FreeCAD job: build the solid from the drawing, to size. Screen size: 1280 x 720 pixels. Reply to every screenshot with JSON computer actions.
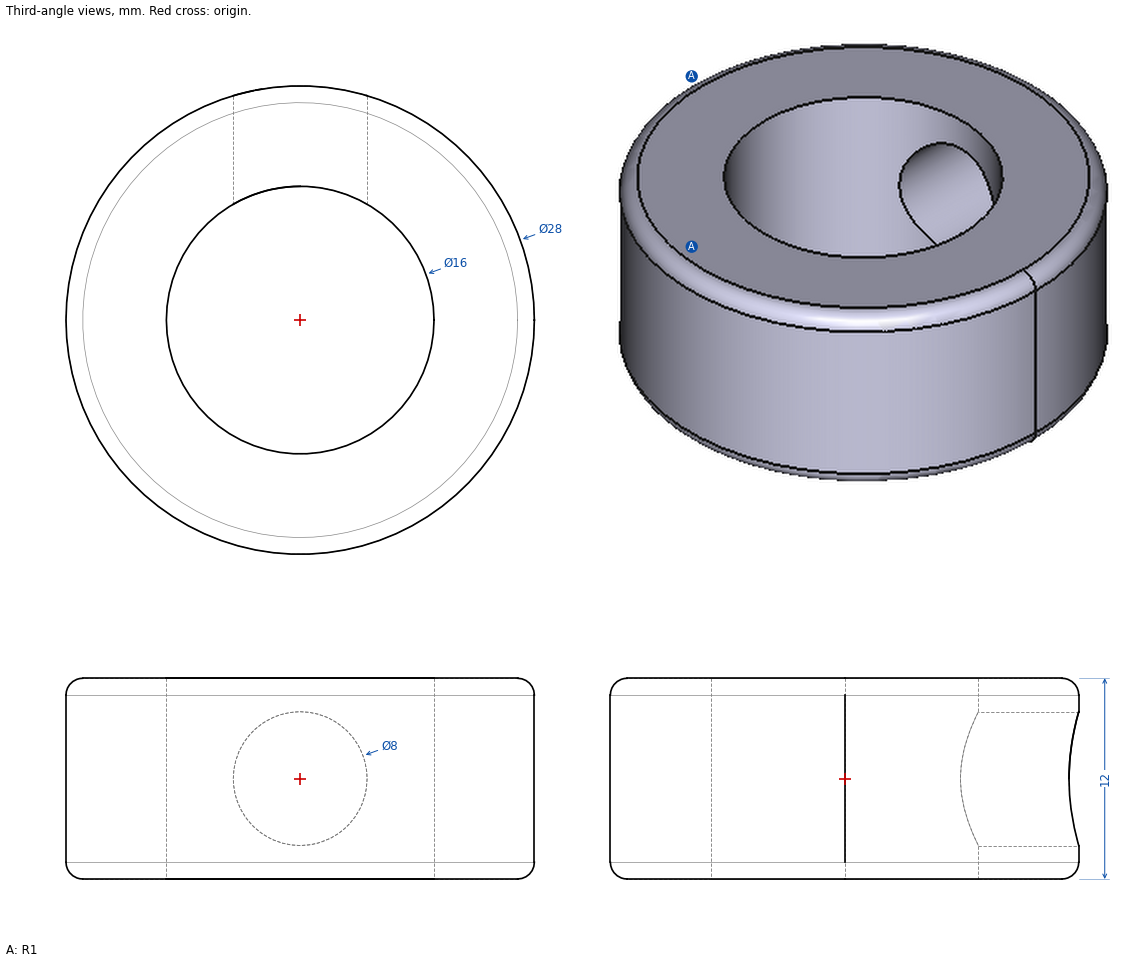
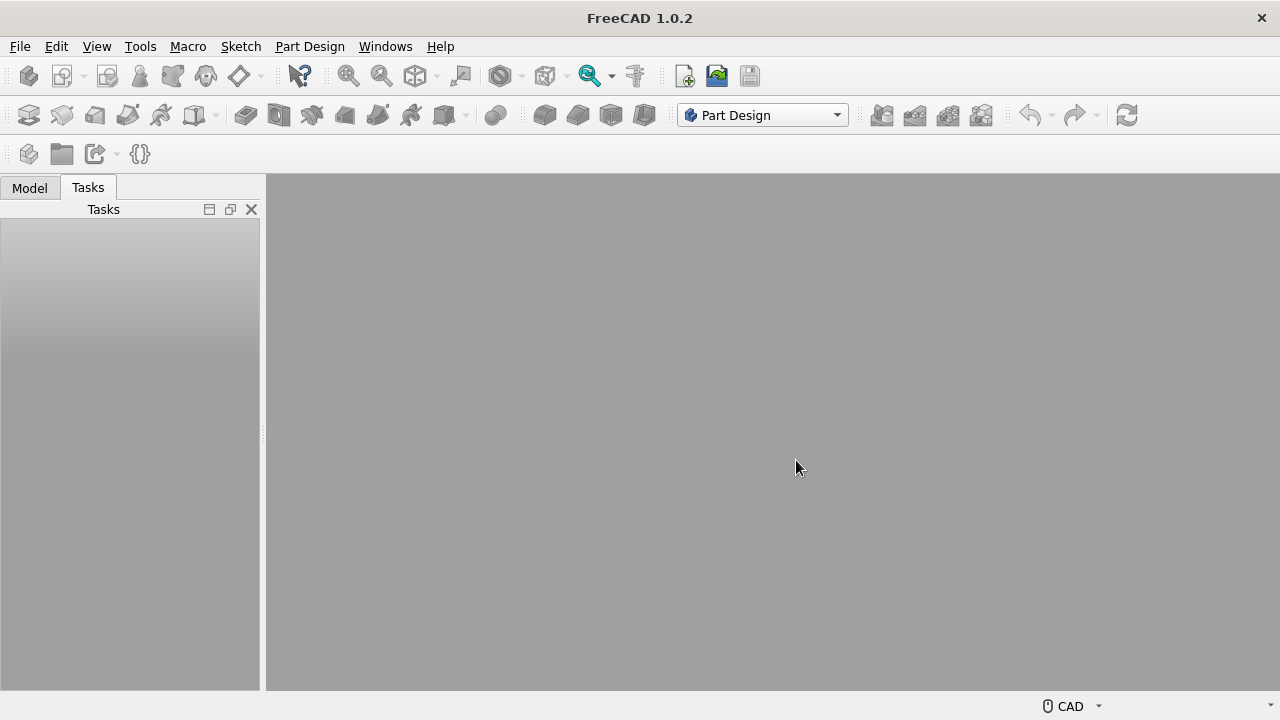
{"action": "key", "text": "ctrl+n"}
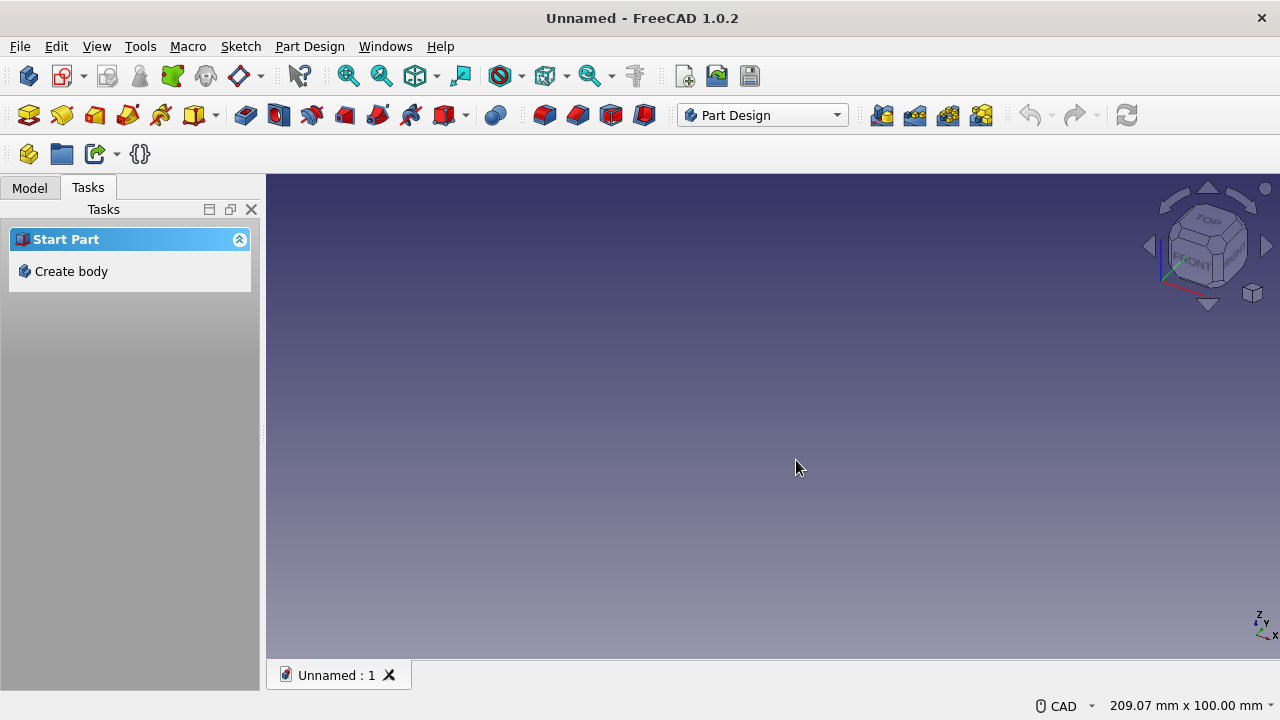
{"action": "left_click", "coordinate": [62, 76]}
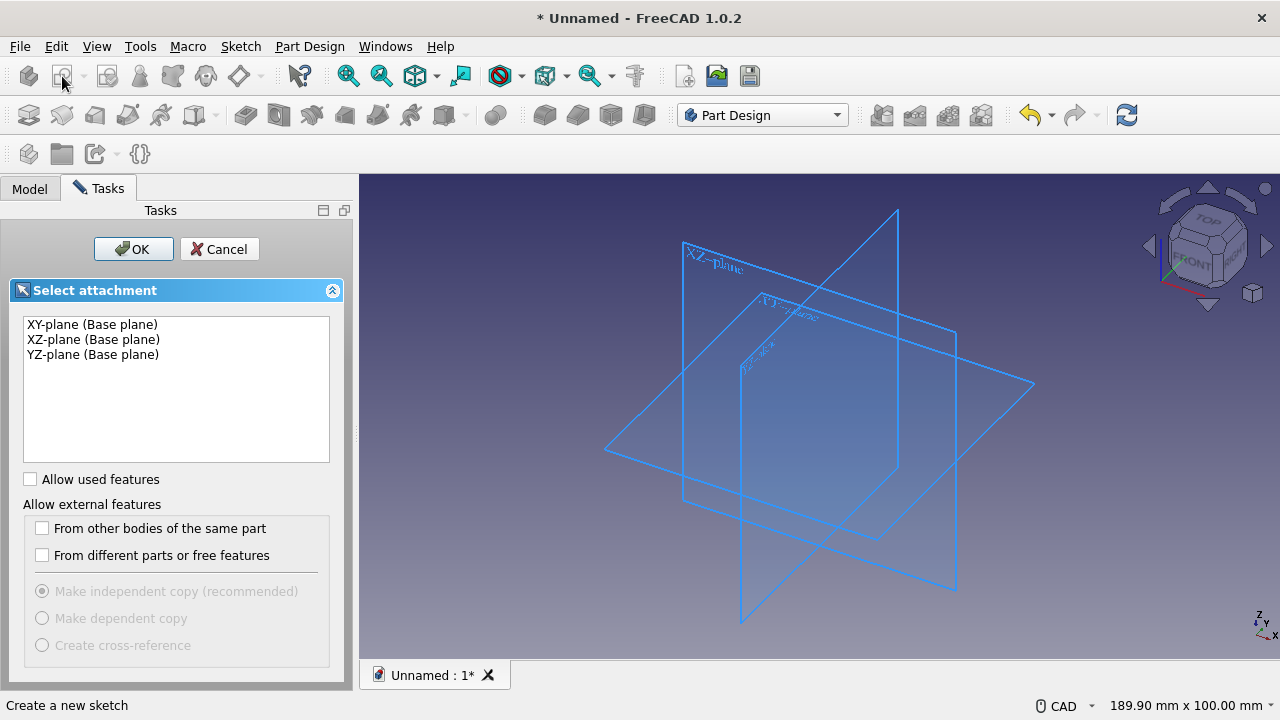
{"action": "left_click", "coordinate": [84, 324]}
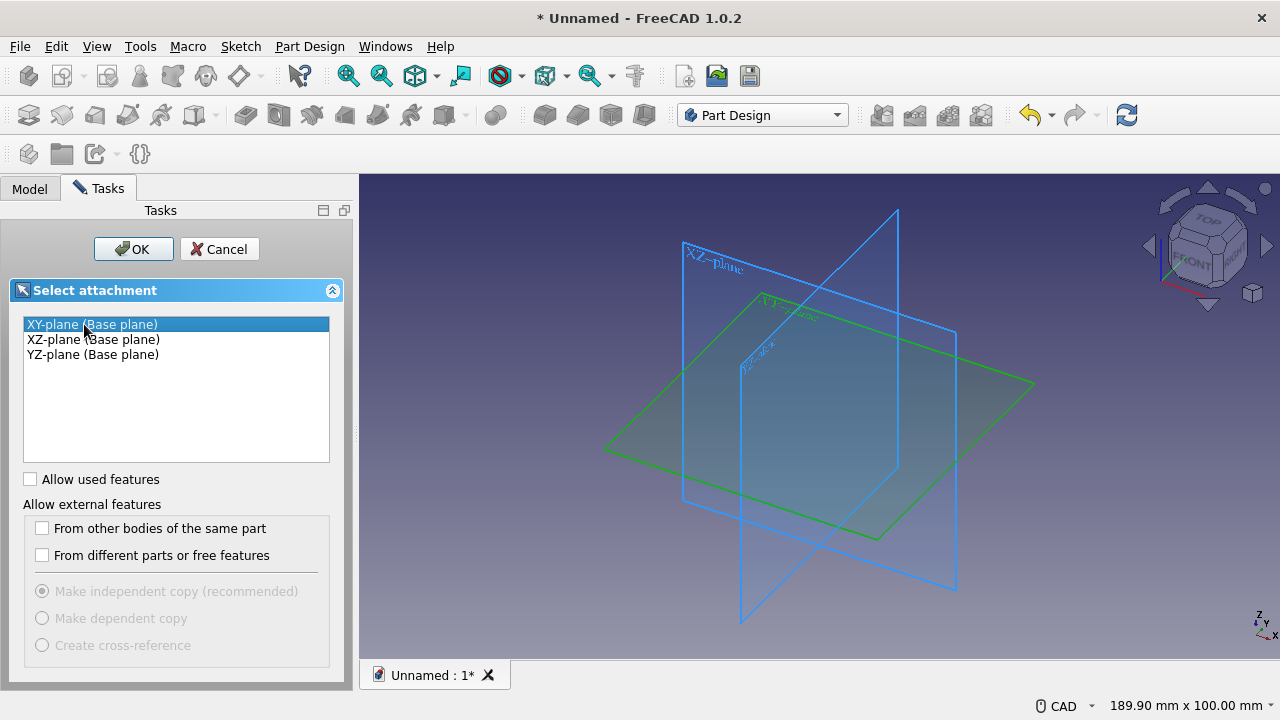
{"action": "left_click", "coordinate": [134, 249]}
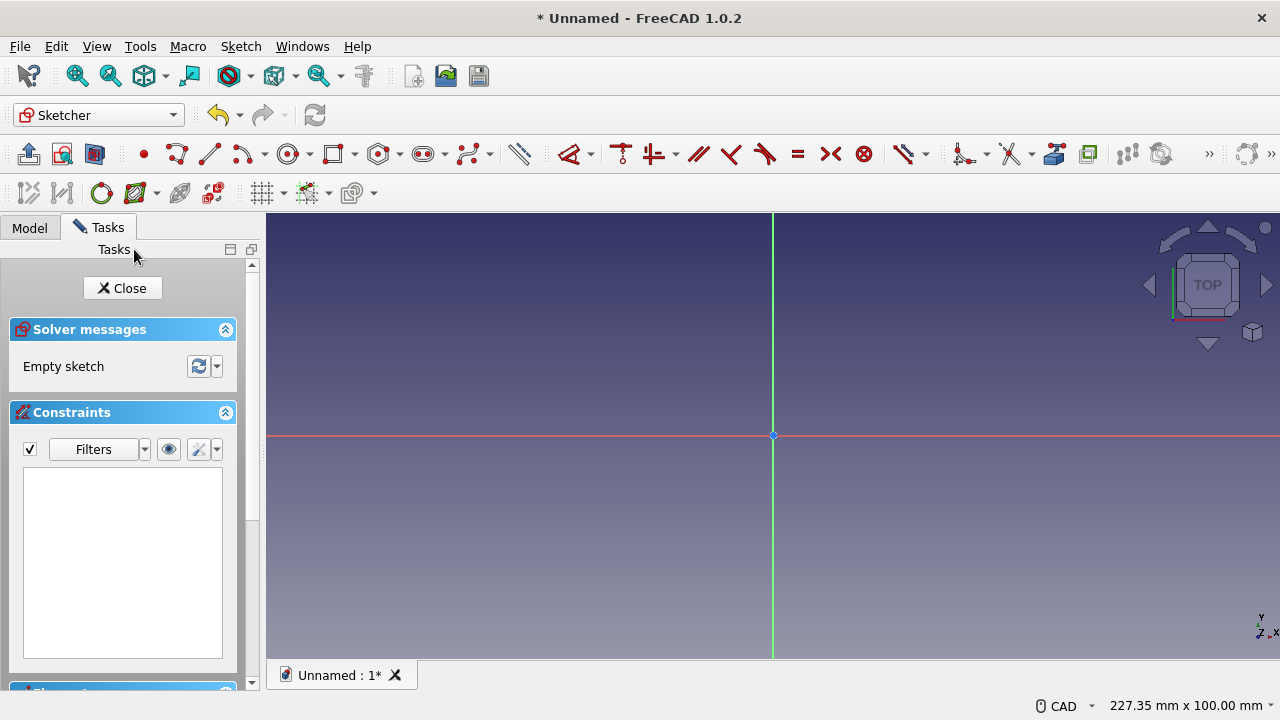
{"action": "scroll", "coordinate": [829, 436], "scroll_direction": "up", "scroll_amount": 4}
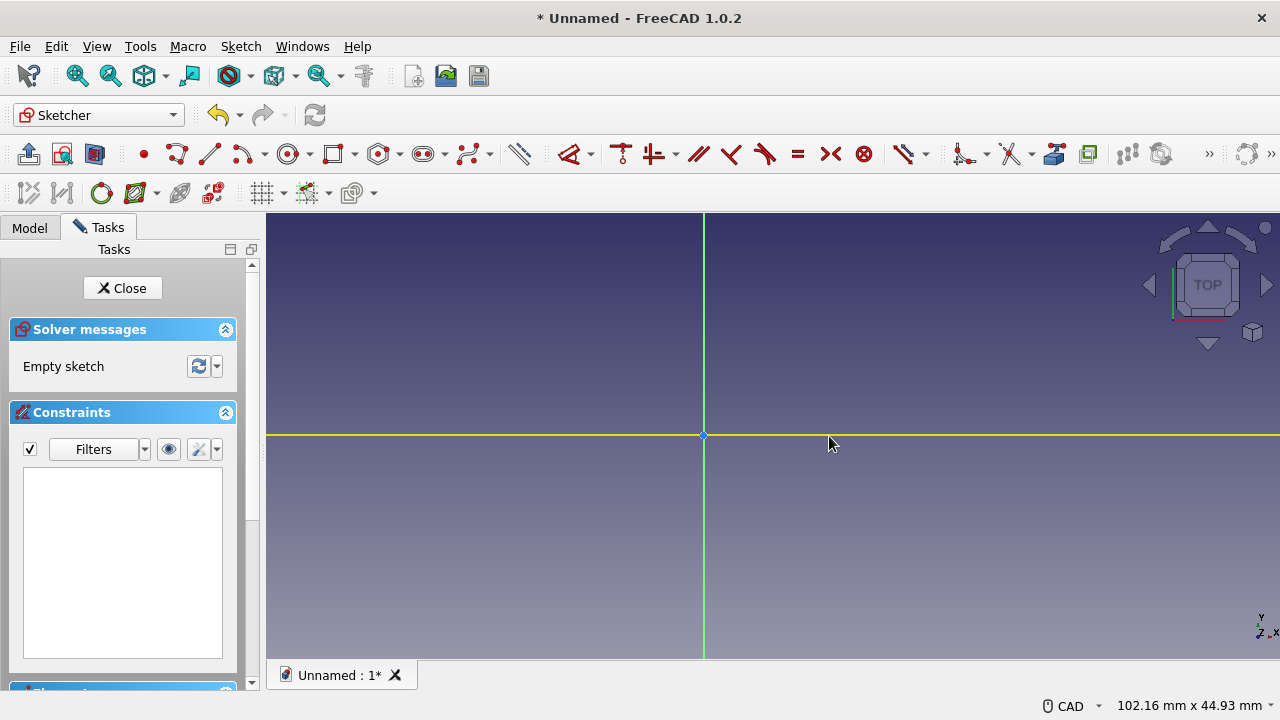
{"action": "key", "text": "g c"}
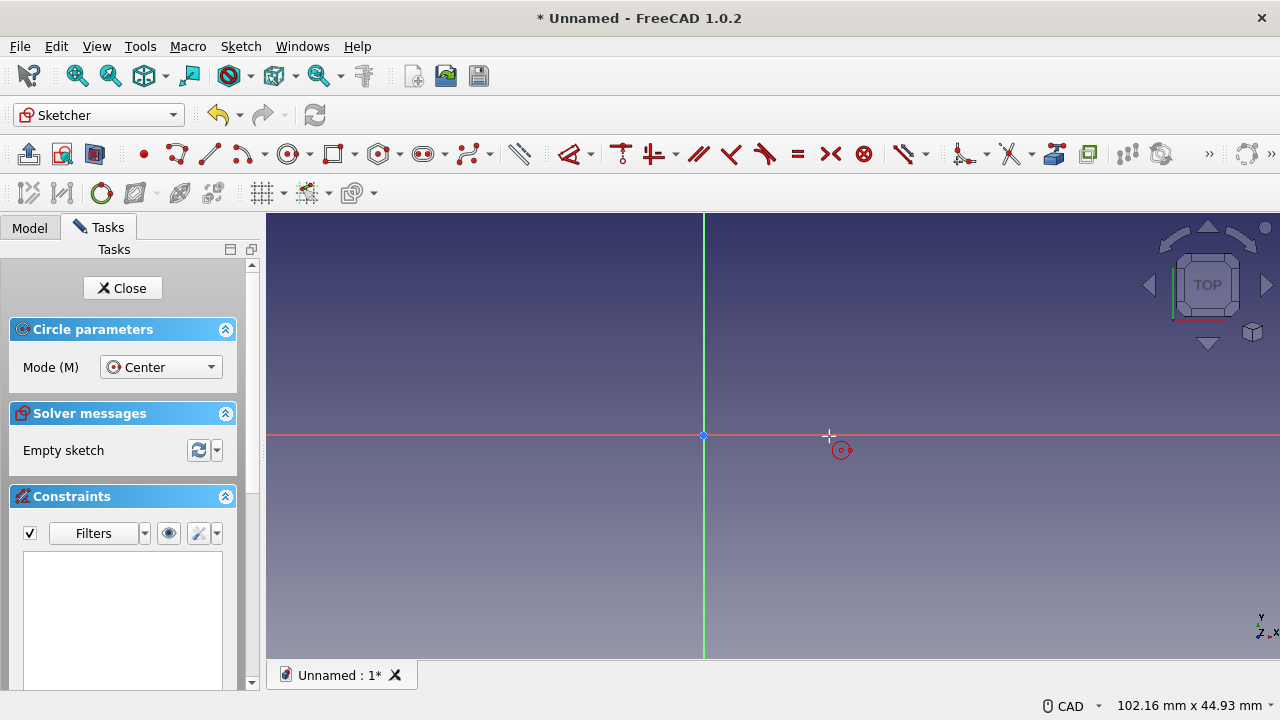
{"action": "left_click", "coordinate": [704, 435]}
{"action": "left_click", "coordinate": [802, 337]}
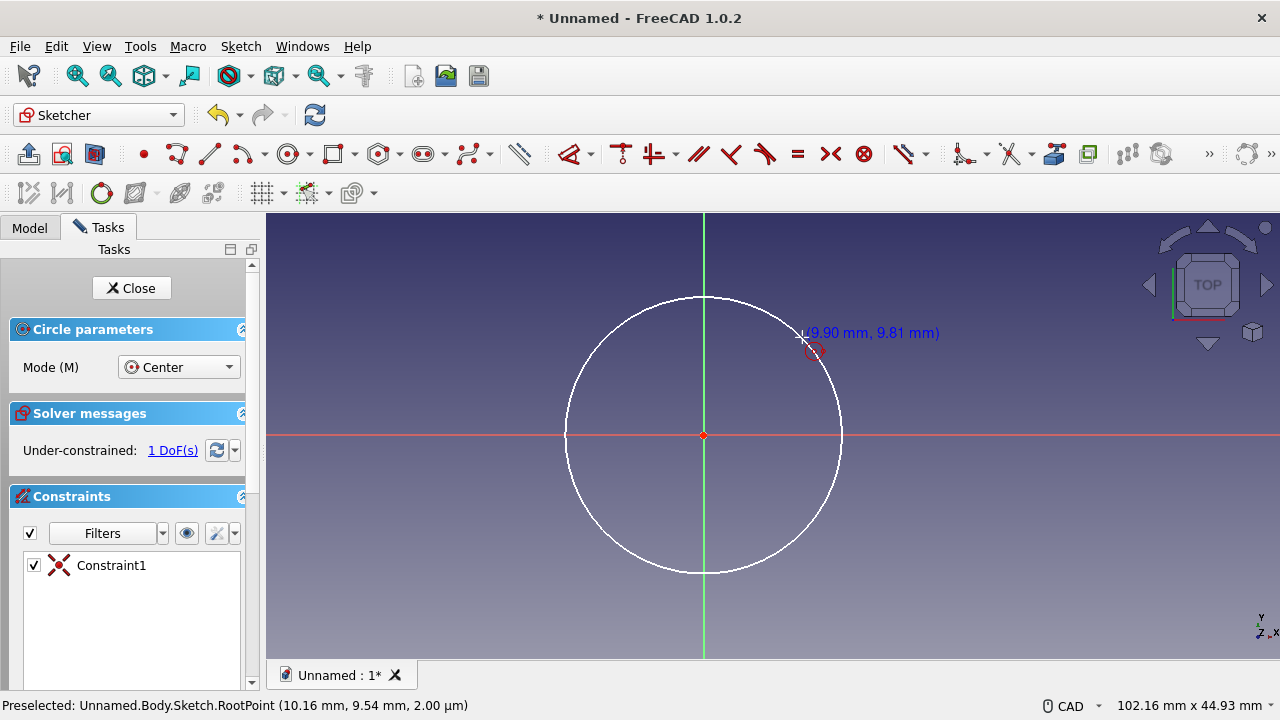
{"action": "left_click", "coordinate": [704, 435]}
{"action": "left_click", "coordinate": [760, 379]}
{"action": "key", "text": "Escape"}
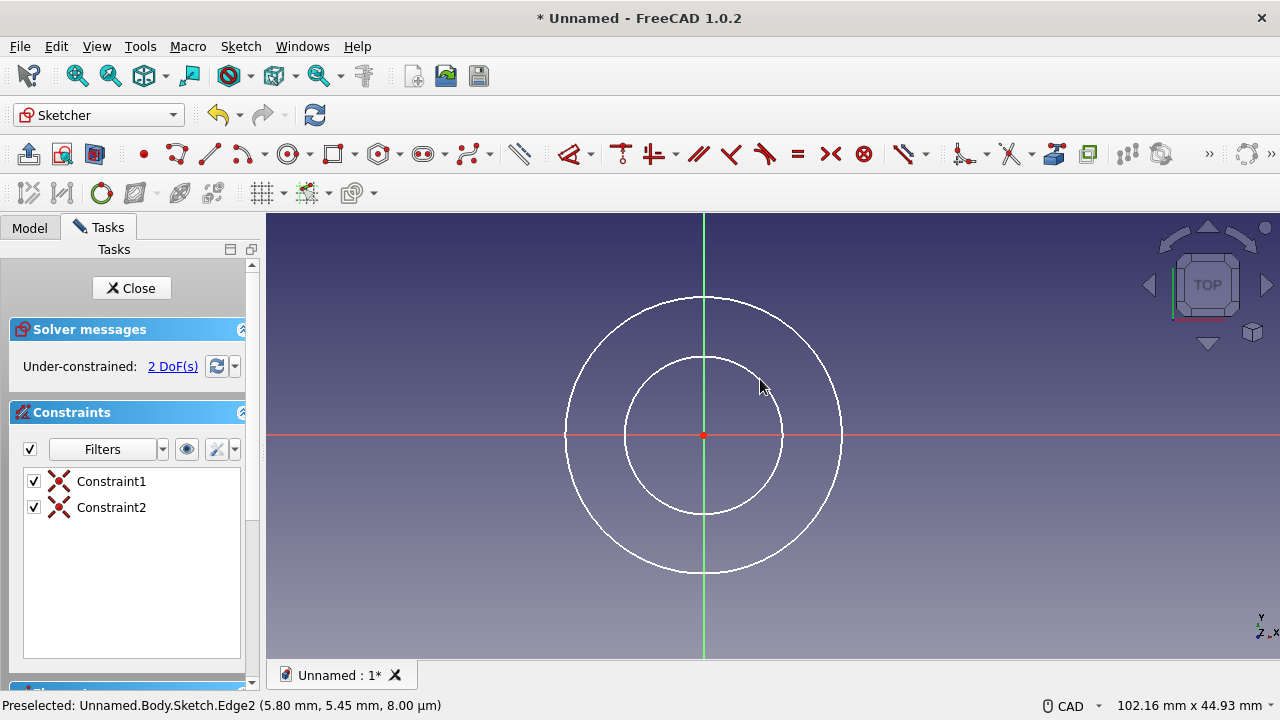
{"action": "left_click", "coordinate": [568, 154]}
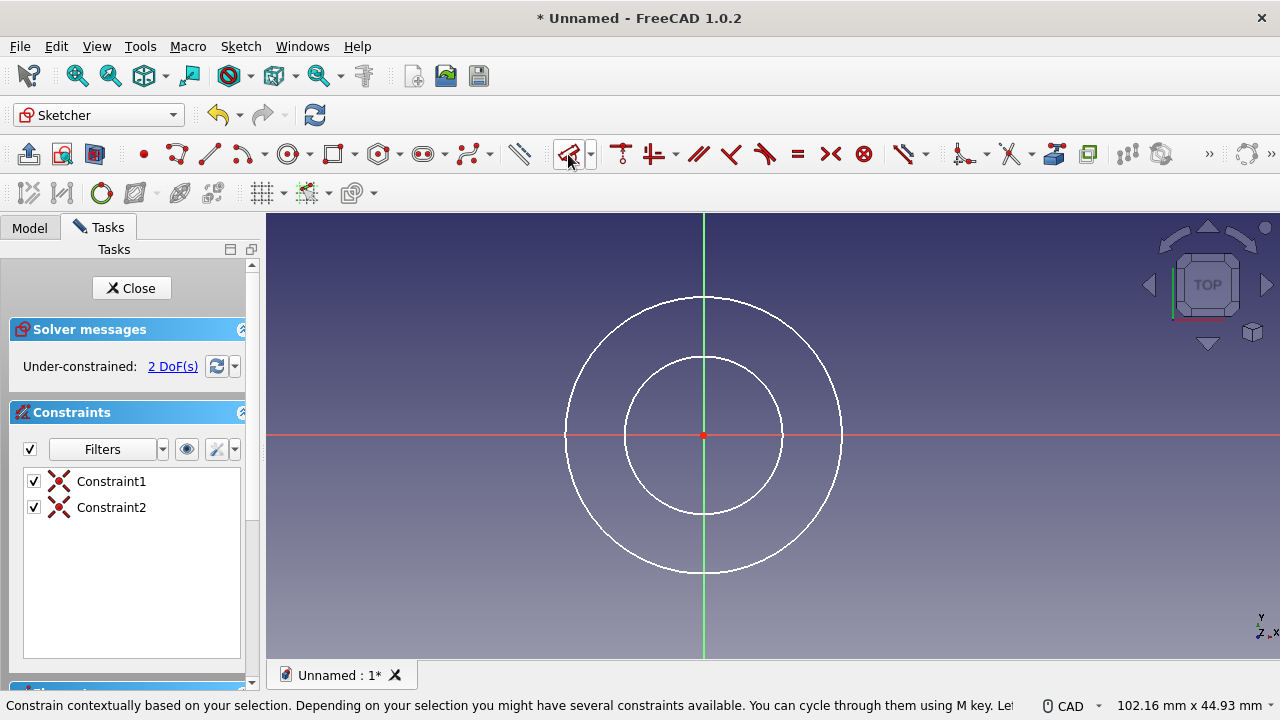
{"action": "left_click", "coordinate": [801, 337]}
{"action": "left_click", "coordinate": [824, 314]}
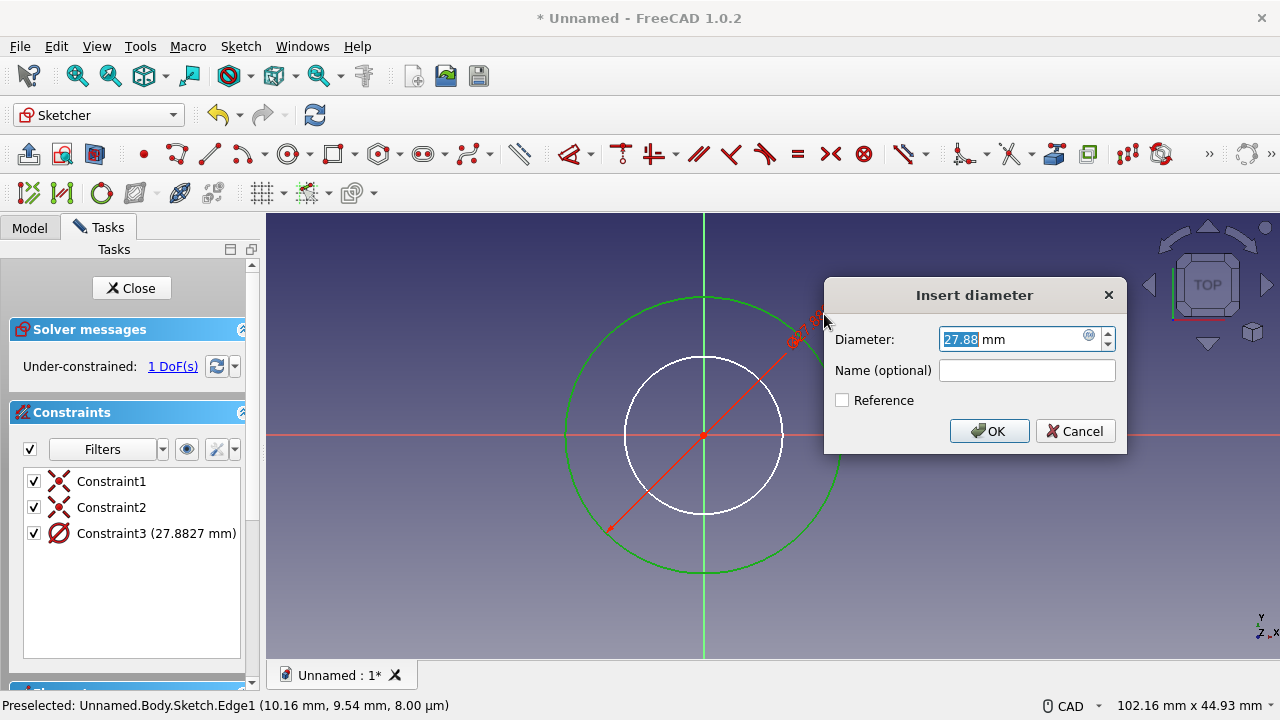
{"action": "type", "text": "28"}
{"action": "key", "text": "Return"}